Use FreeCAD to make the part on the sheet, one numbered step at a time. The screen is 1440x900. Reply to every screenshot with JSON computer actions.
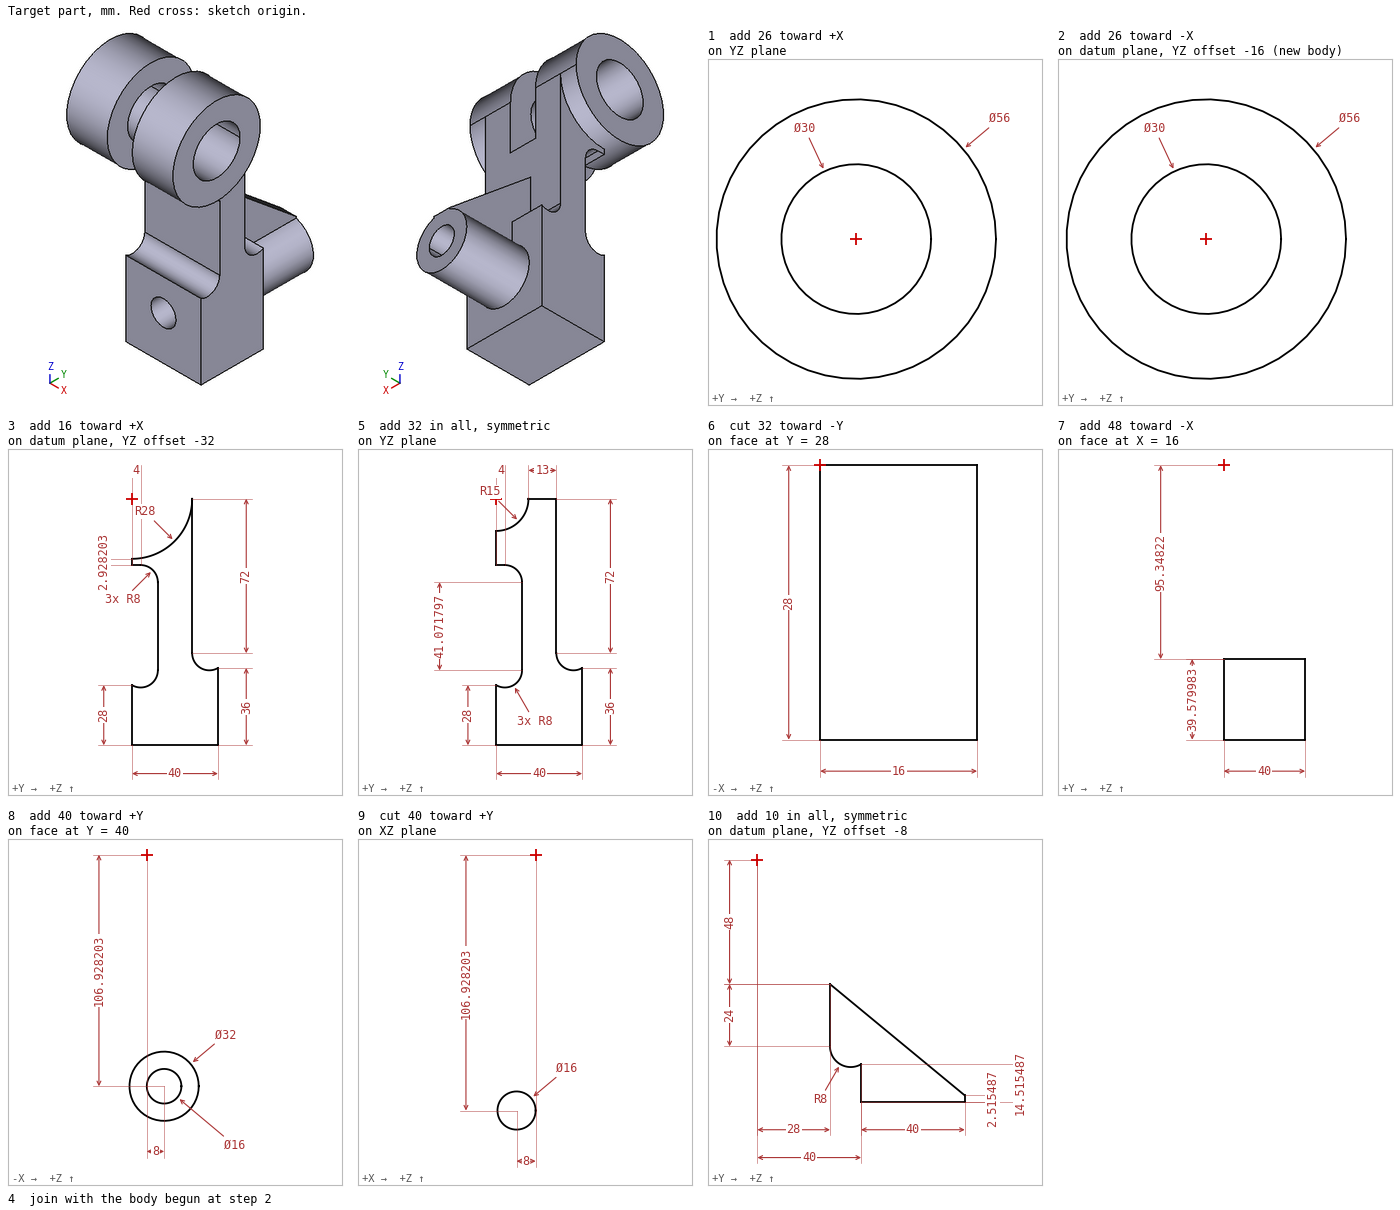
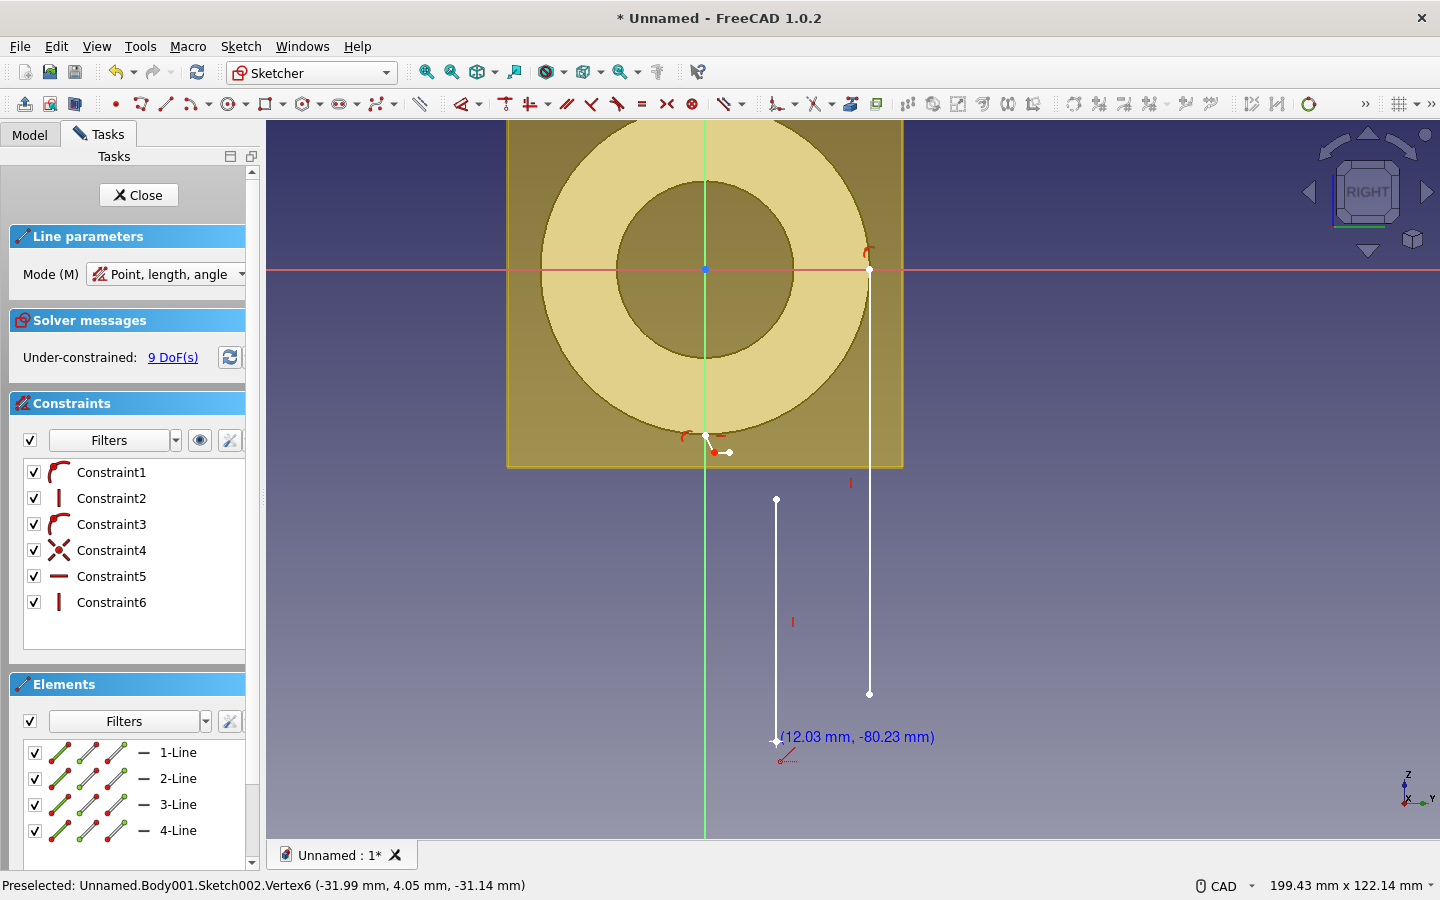
{"action": "key", "text": "g m"}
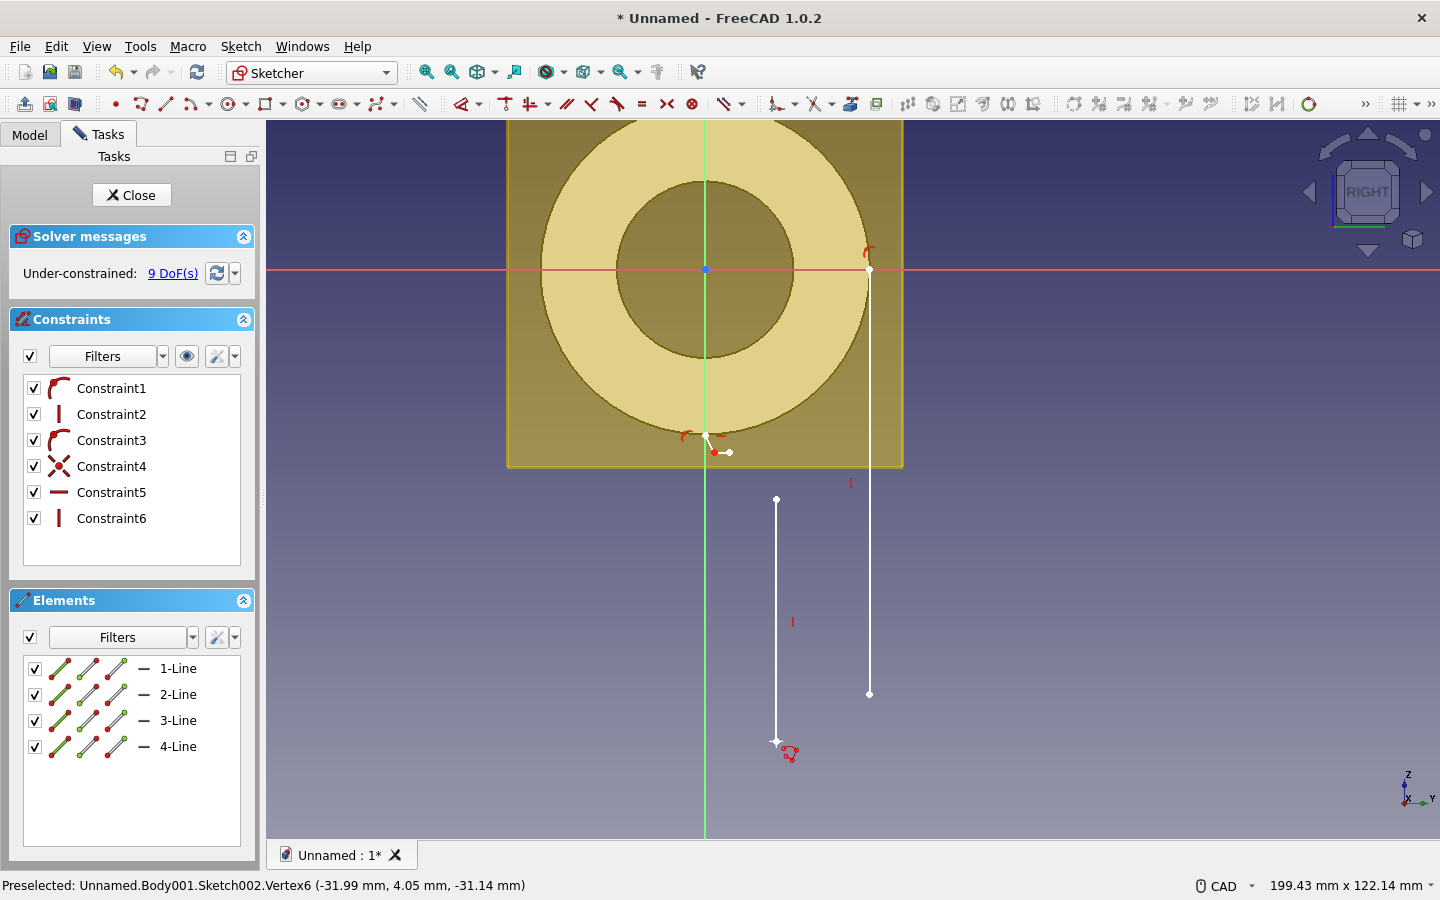
{"action": "left_click", "coordinate": [705, 781]}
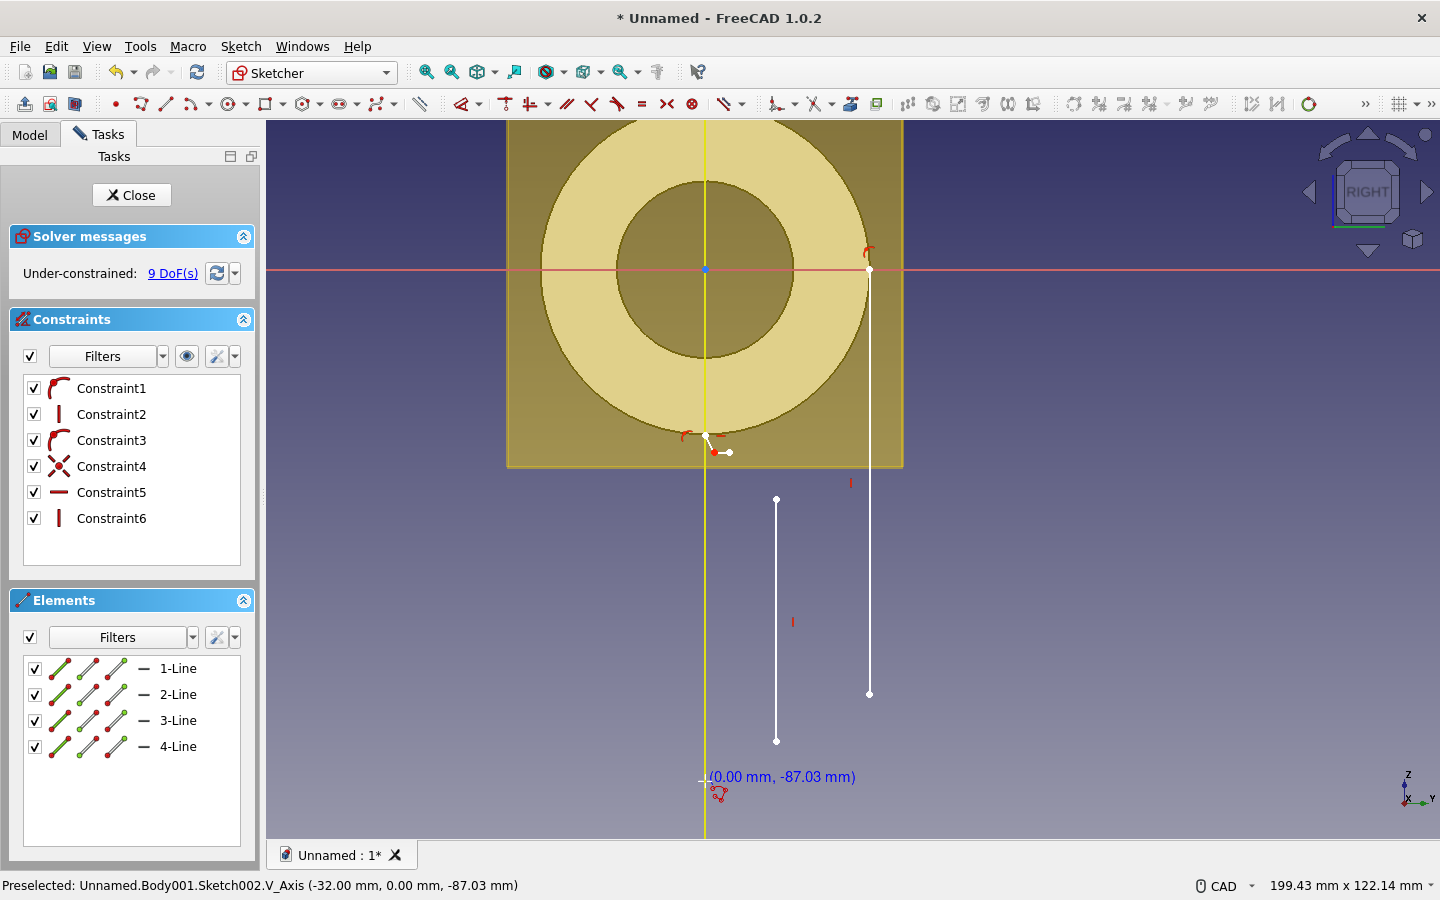
{"action": "scroll", "coordinate": [706, 218], "scroll_direction": "down", "scroll_amount": 2}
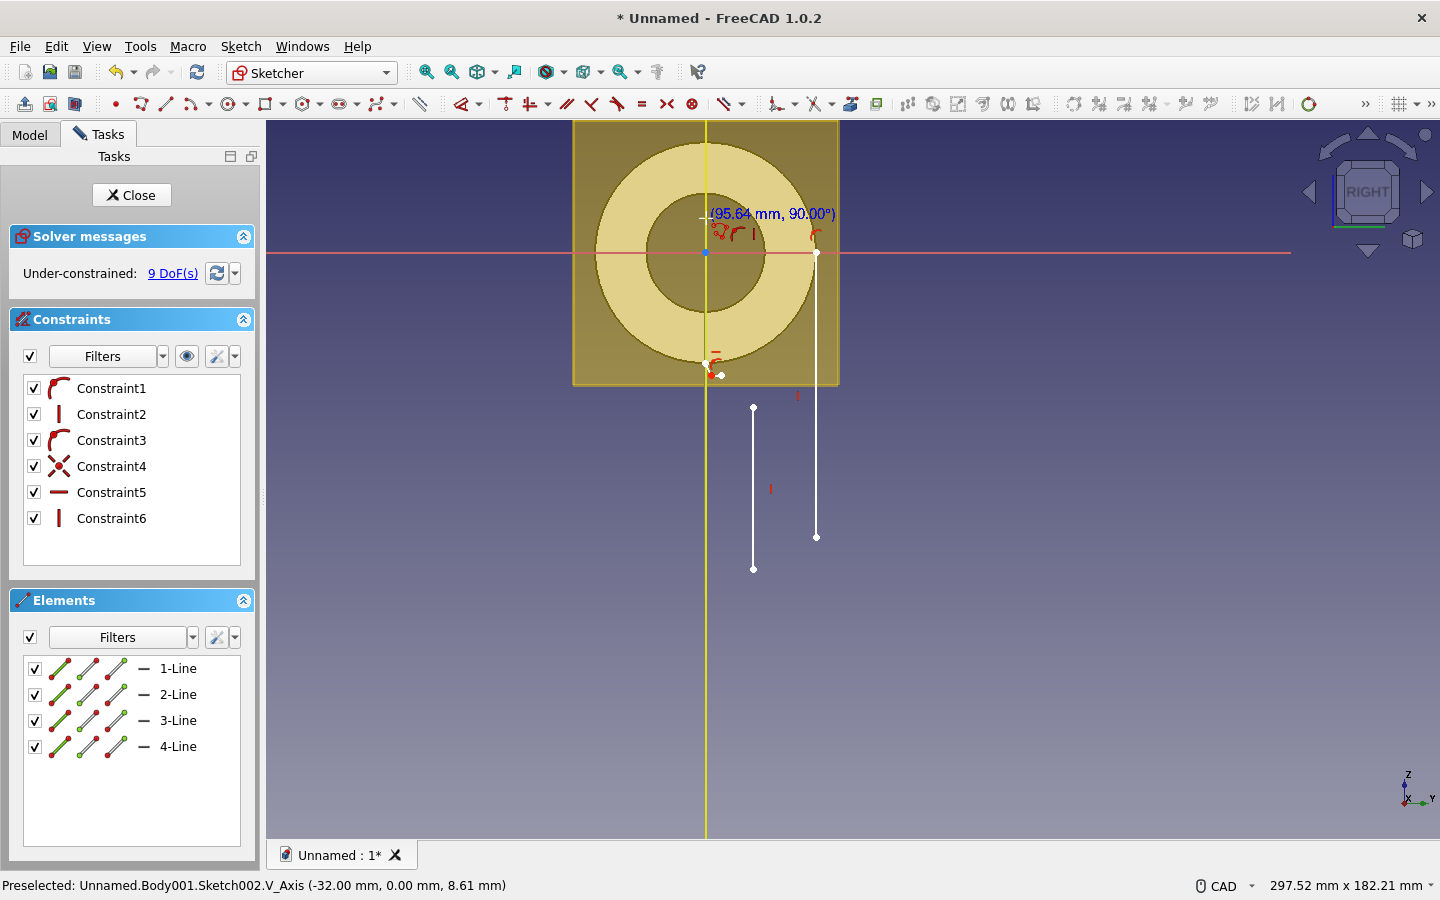
{"action": "left_click", "coordinate": [715, 706]}
{"action": "left_click", "coordinate": [863, 706]}
{"action": "left_click", "coordinate": [863, 564]}
{"action": "right_click", "coordinate": [863, 564]}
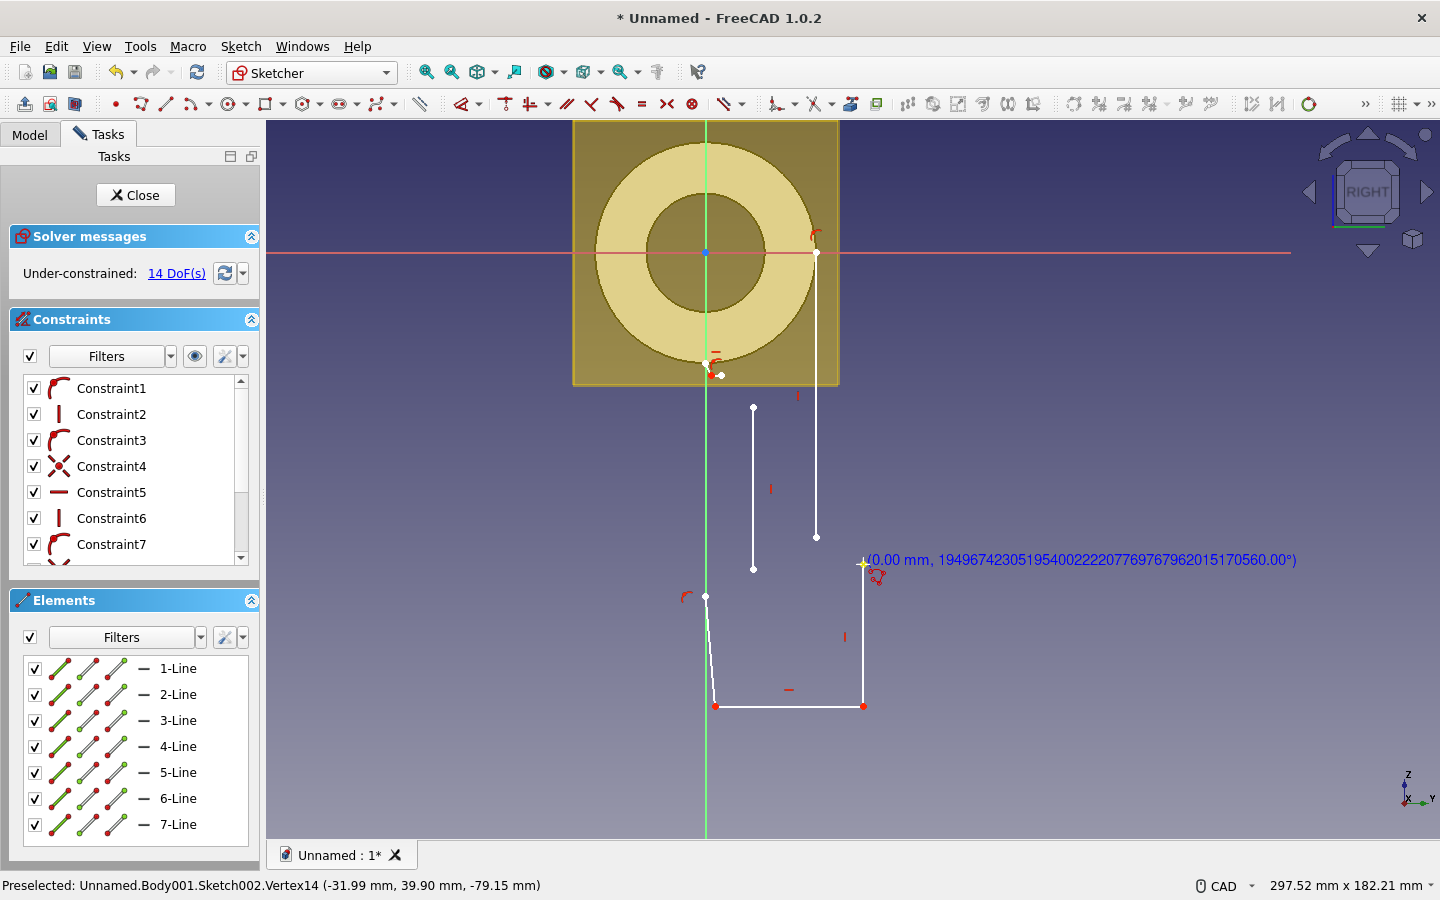
{"action": "left_click", "coordinate": [208, 104]}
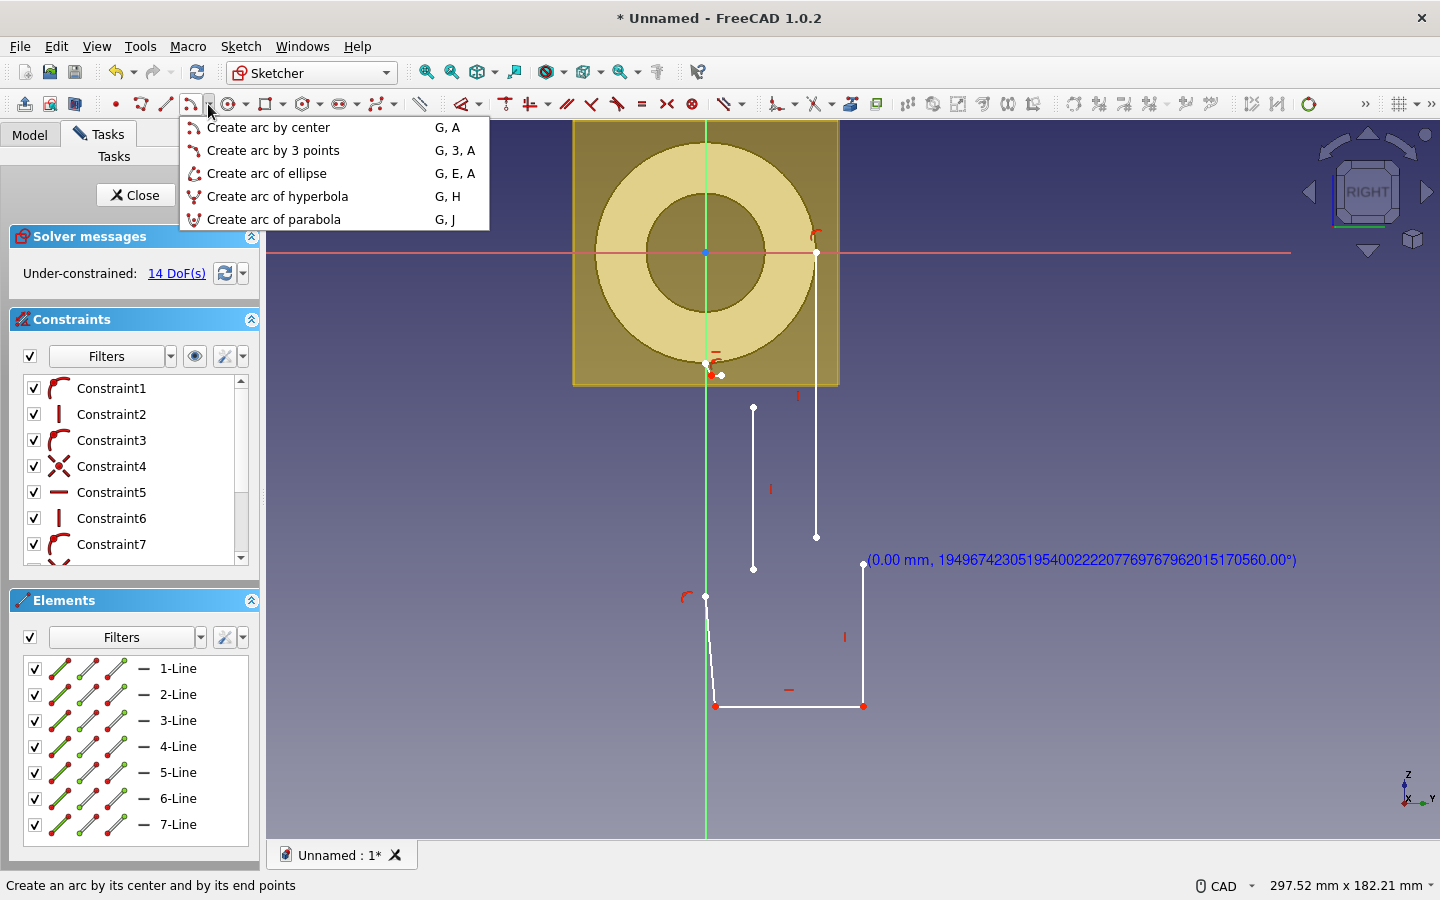
{"action": "left_click", "coordinate": [334, 150]}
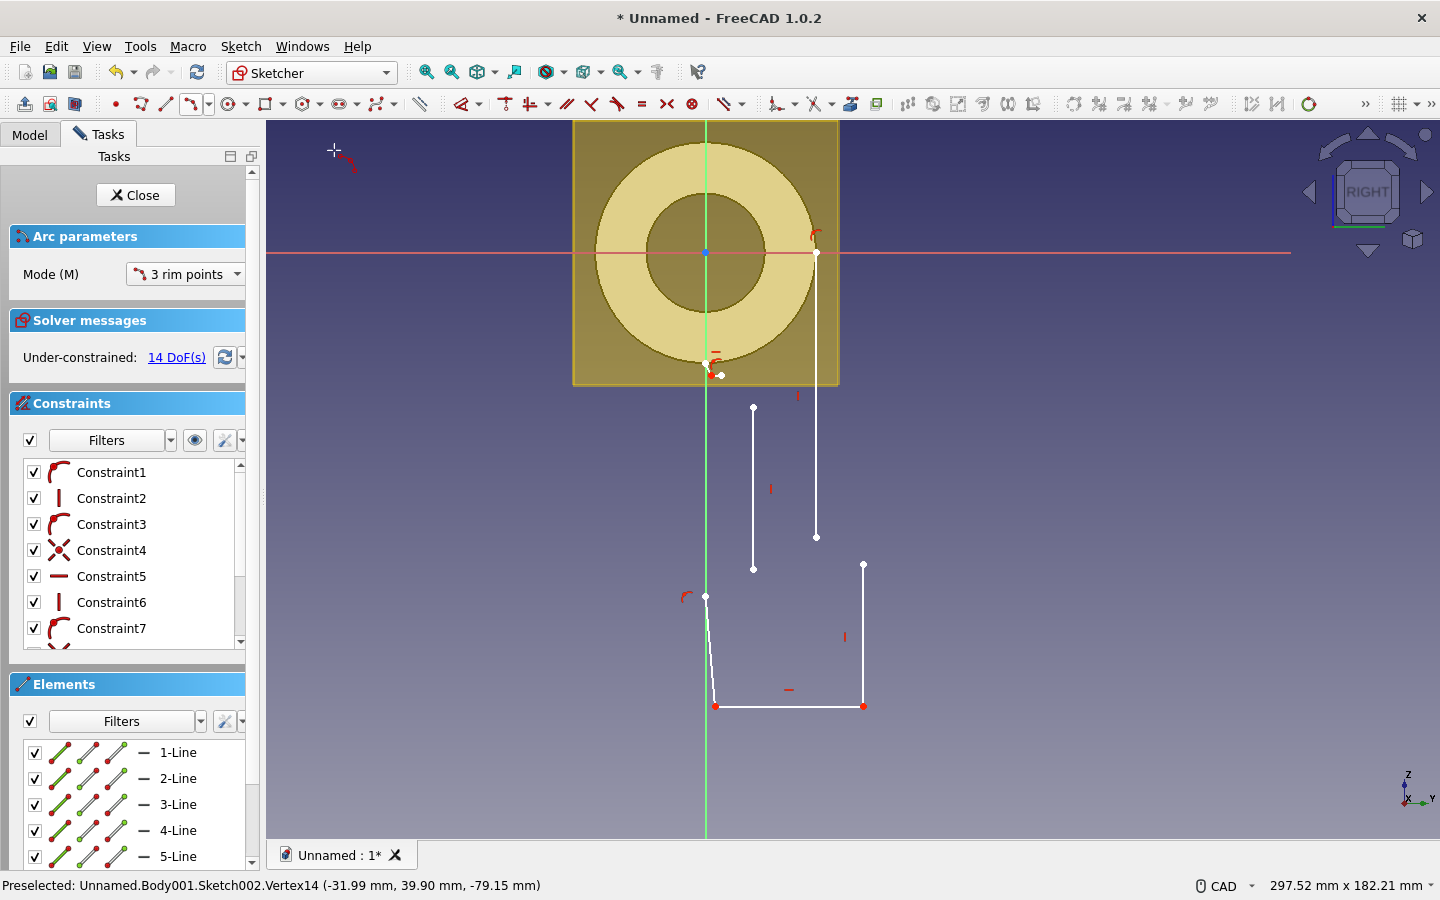
{"action": "left_click", "coordinate": [816, 253]}